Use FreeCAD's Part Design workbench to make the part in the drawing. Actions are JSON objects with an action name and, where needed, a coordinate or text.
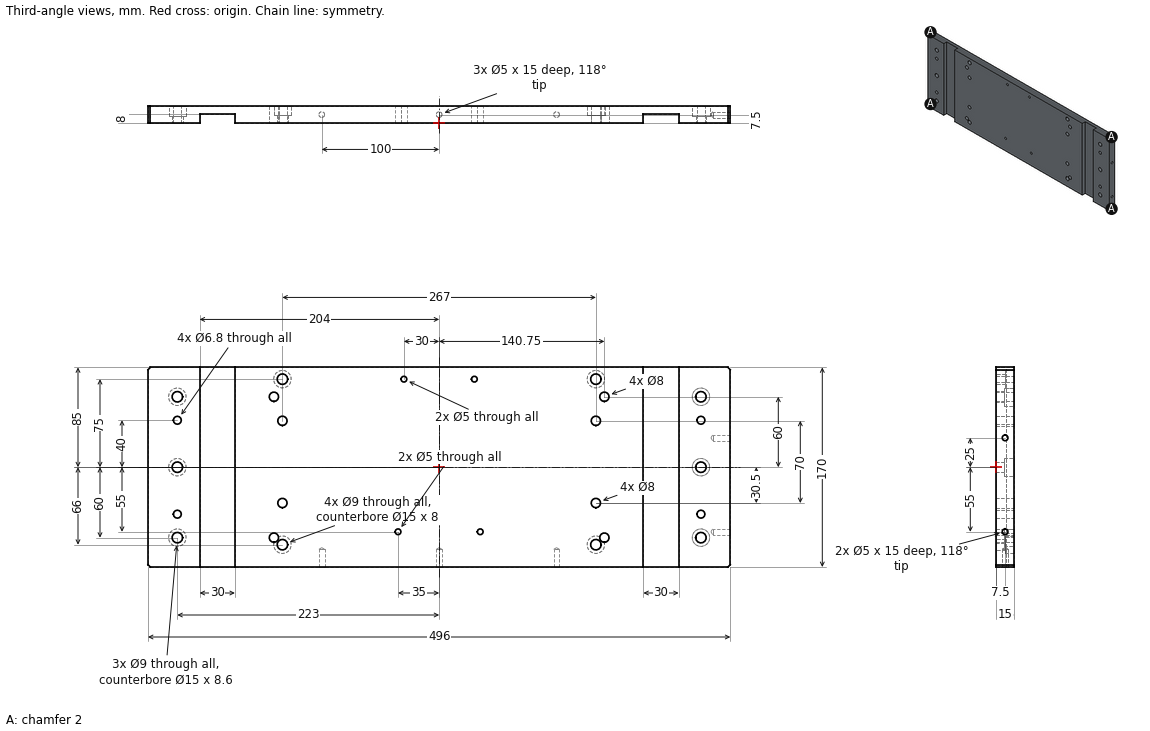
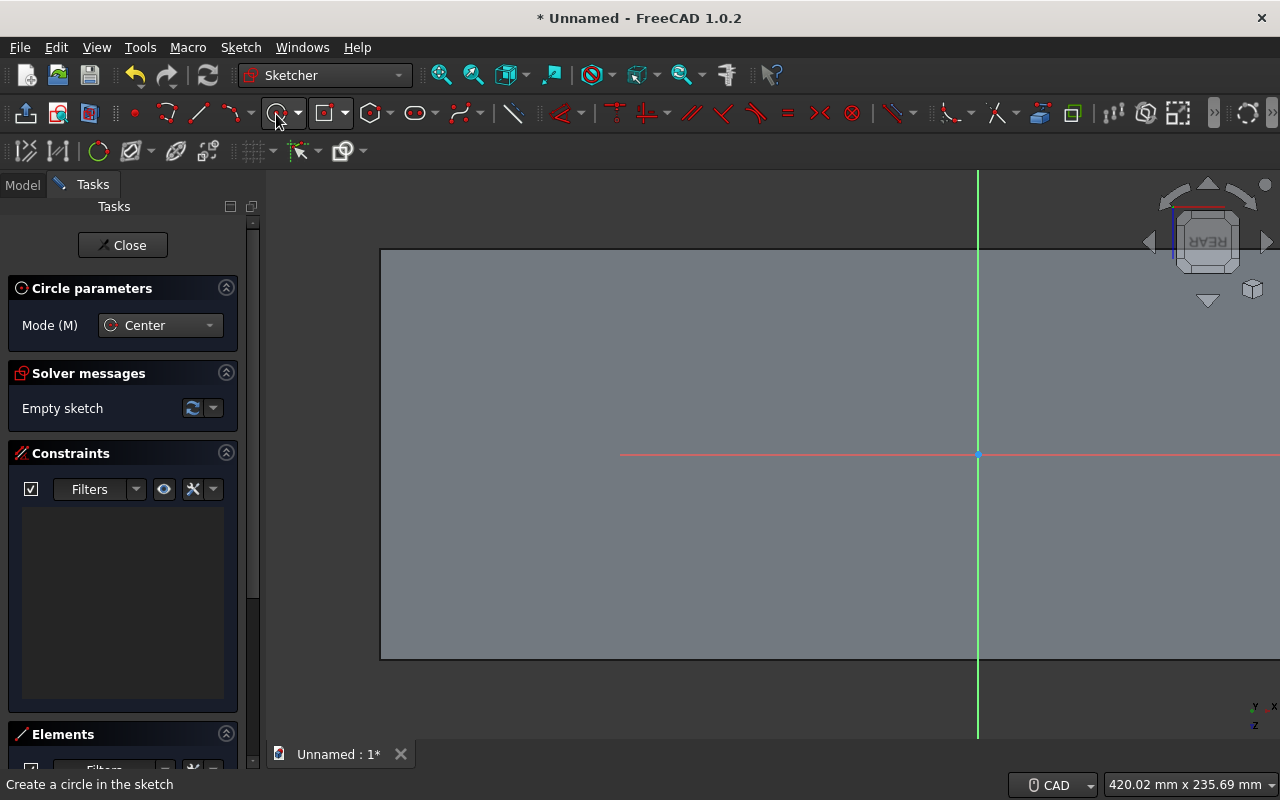
{"action": "scroll", "coordinate": [440, 310], "scroll_direction": "up", "scroll_amount": 4}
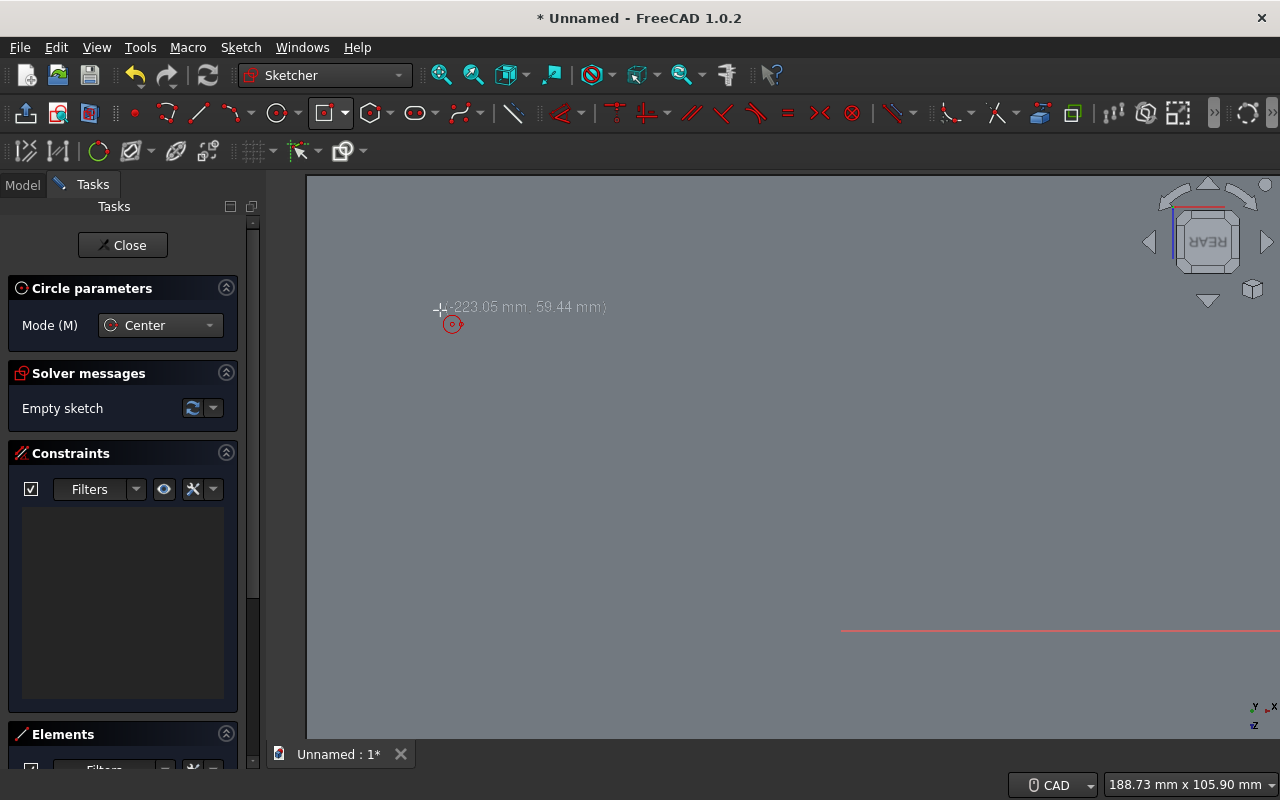
{"action": "left_click", "coordinate": [440, 309]}
{"action": "mouse_move", "coordinate": [457, 292]}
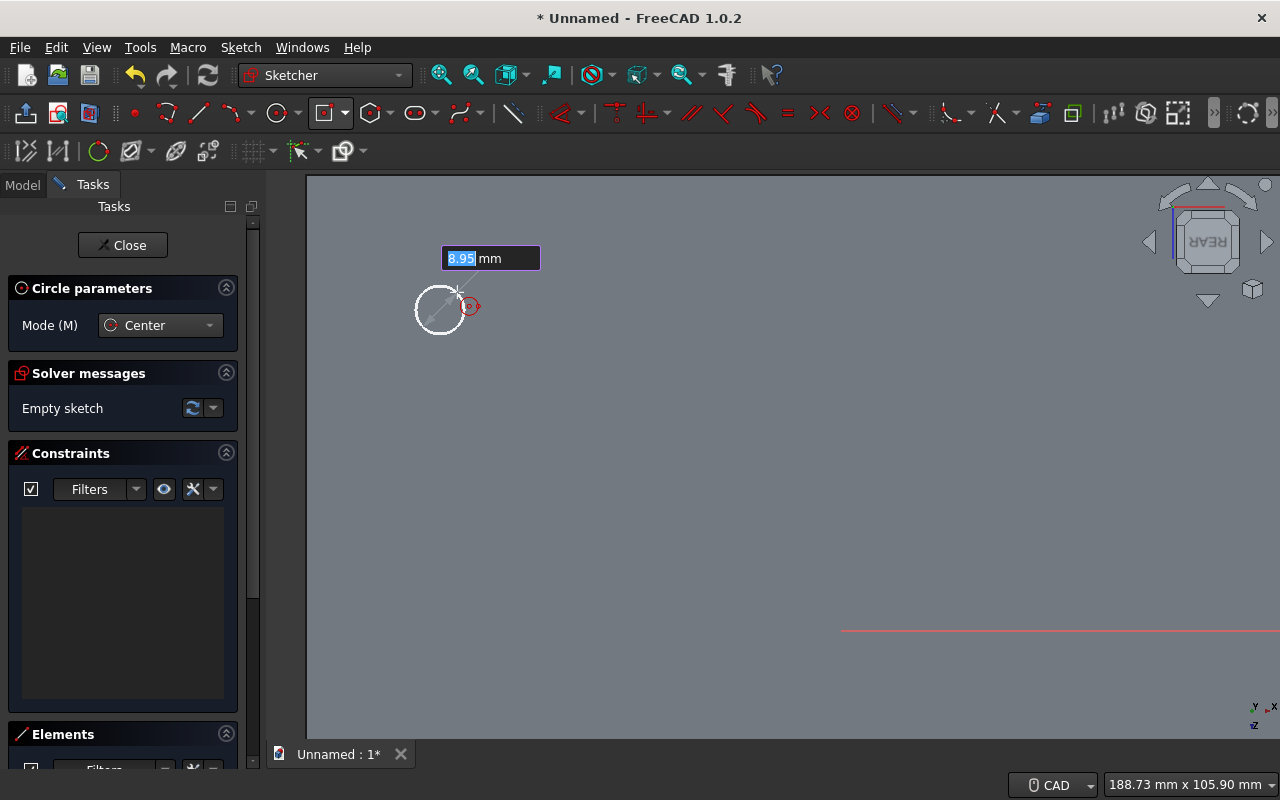
{"action": "type", "text": "9"}
{"action": "key", "text": "Return"}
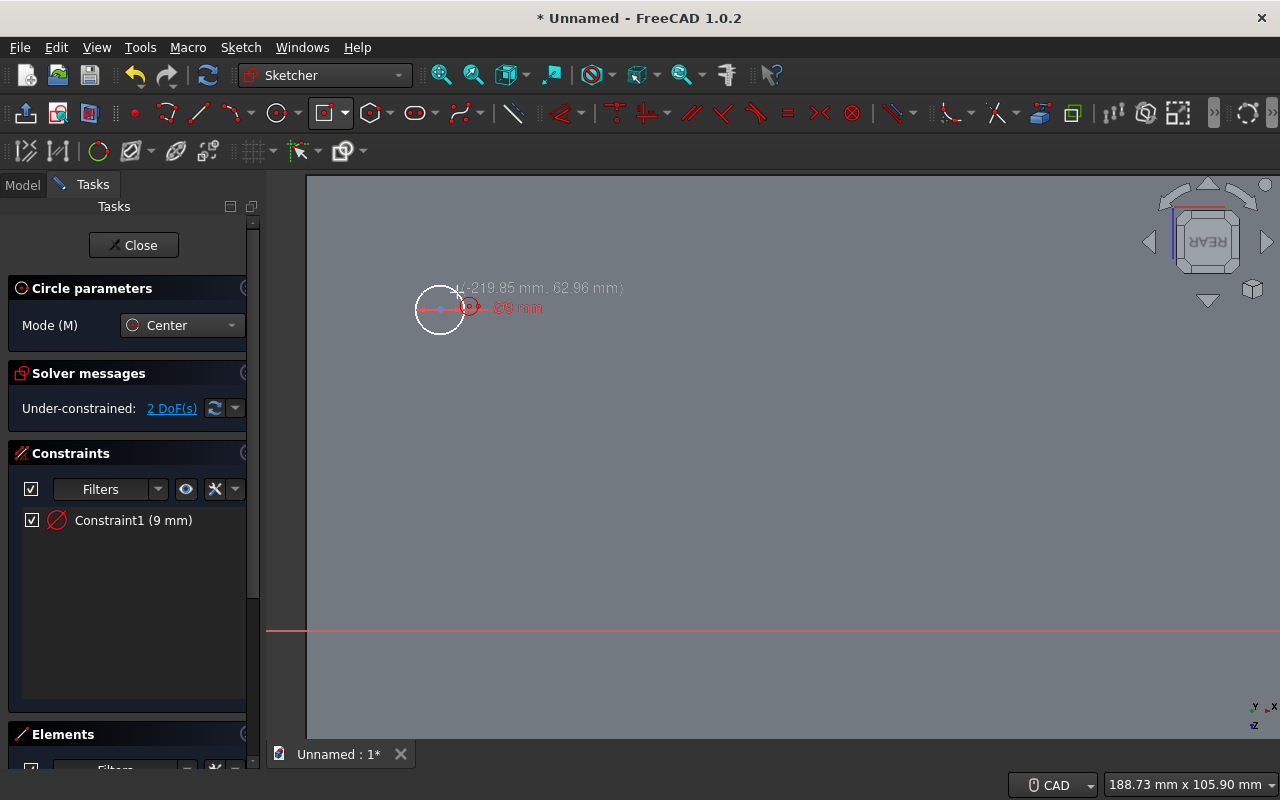
{"action": "left_click", "coordinate": [440, 631]}
{"action": "mouse_move", "coordinate": [457, 614]}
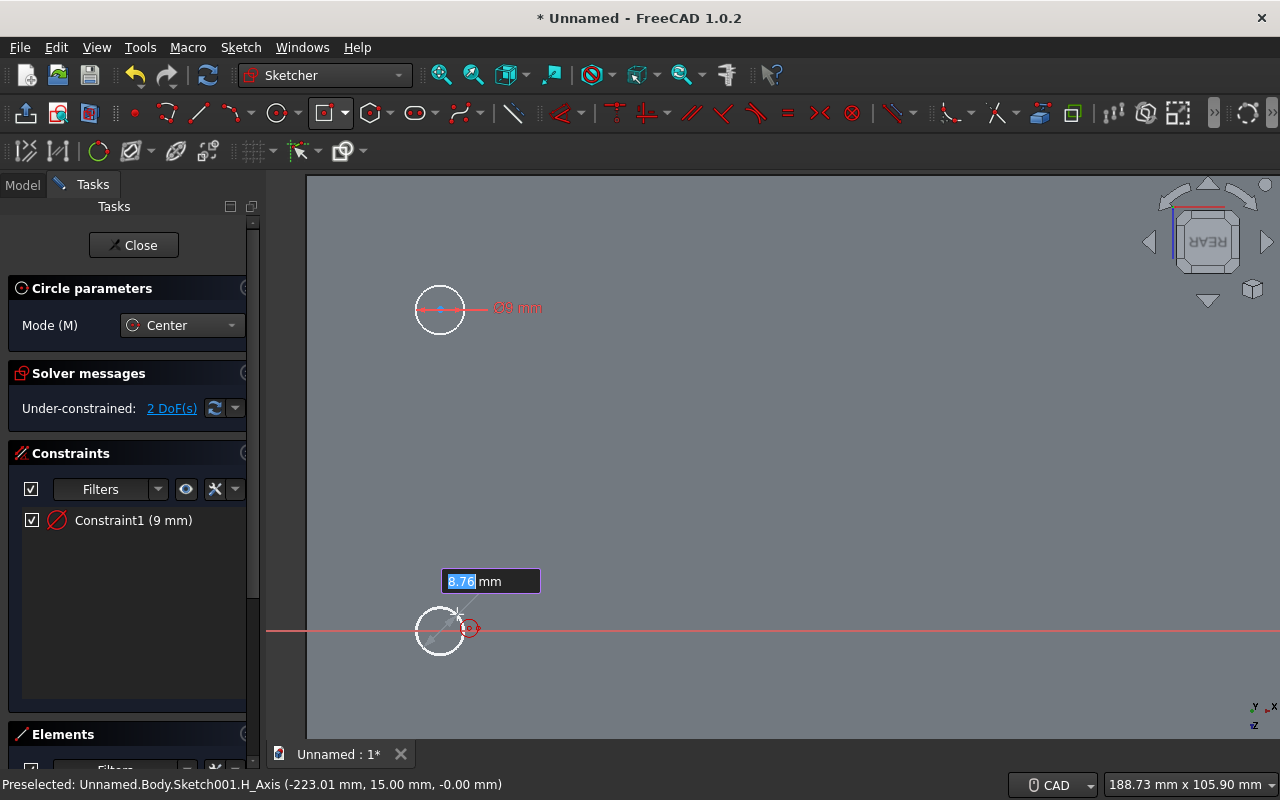
{"action": "type", "text": "9"}
{"action": "key", "text": "Return"}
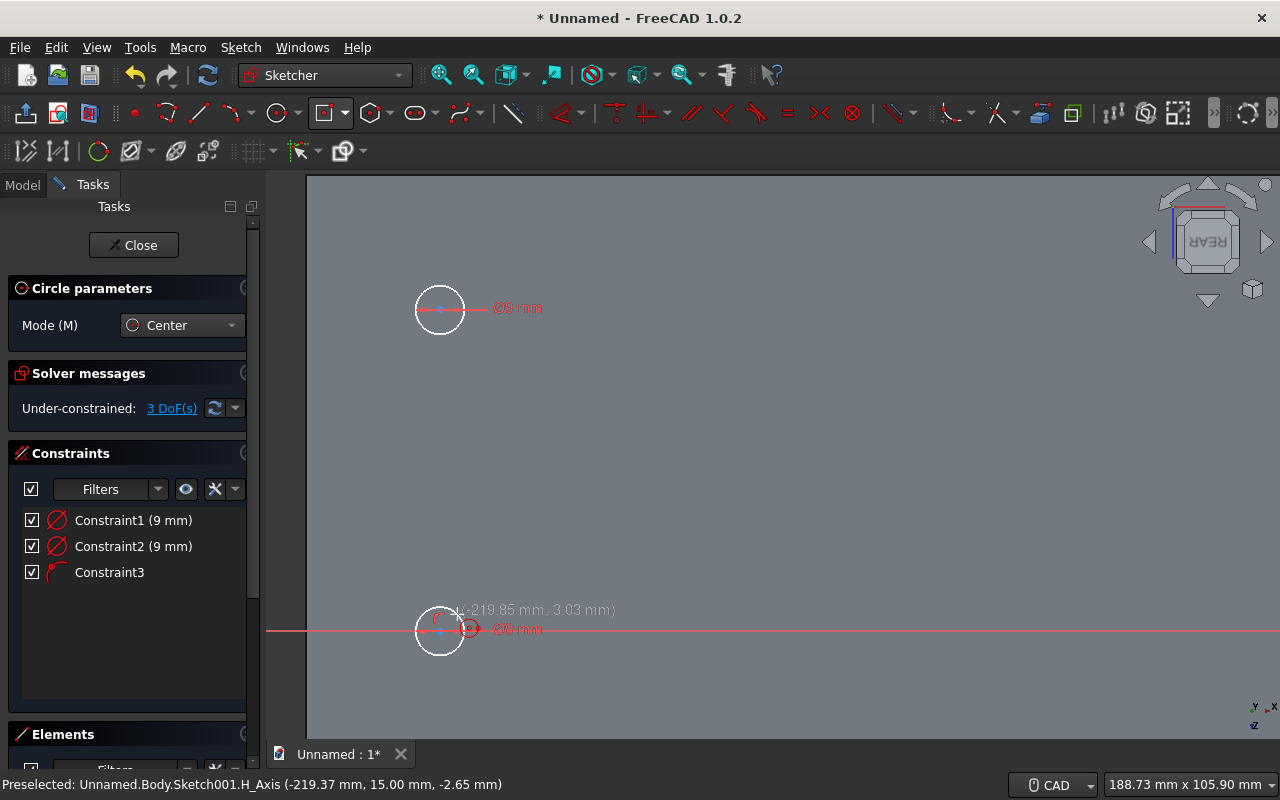
{"action": "scroll", "coordinate": [441, 310], "scroll_direction": "down", "scroll_amount": 4}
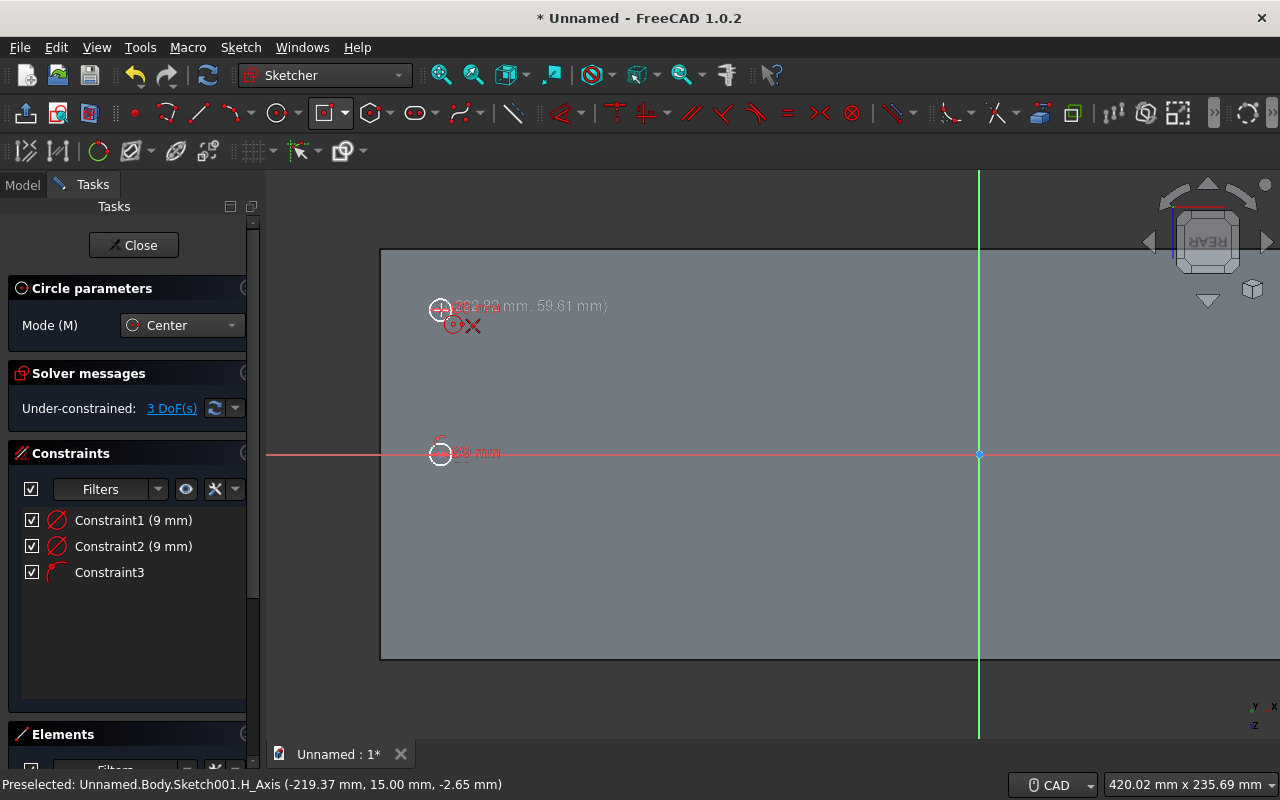
{"action": "scroll", "coordinate": [441, 599], "scroll_direction": "up", "scroll_amount": 4}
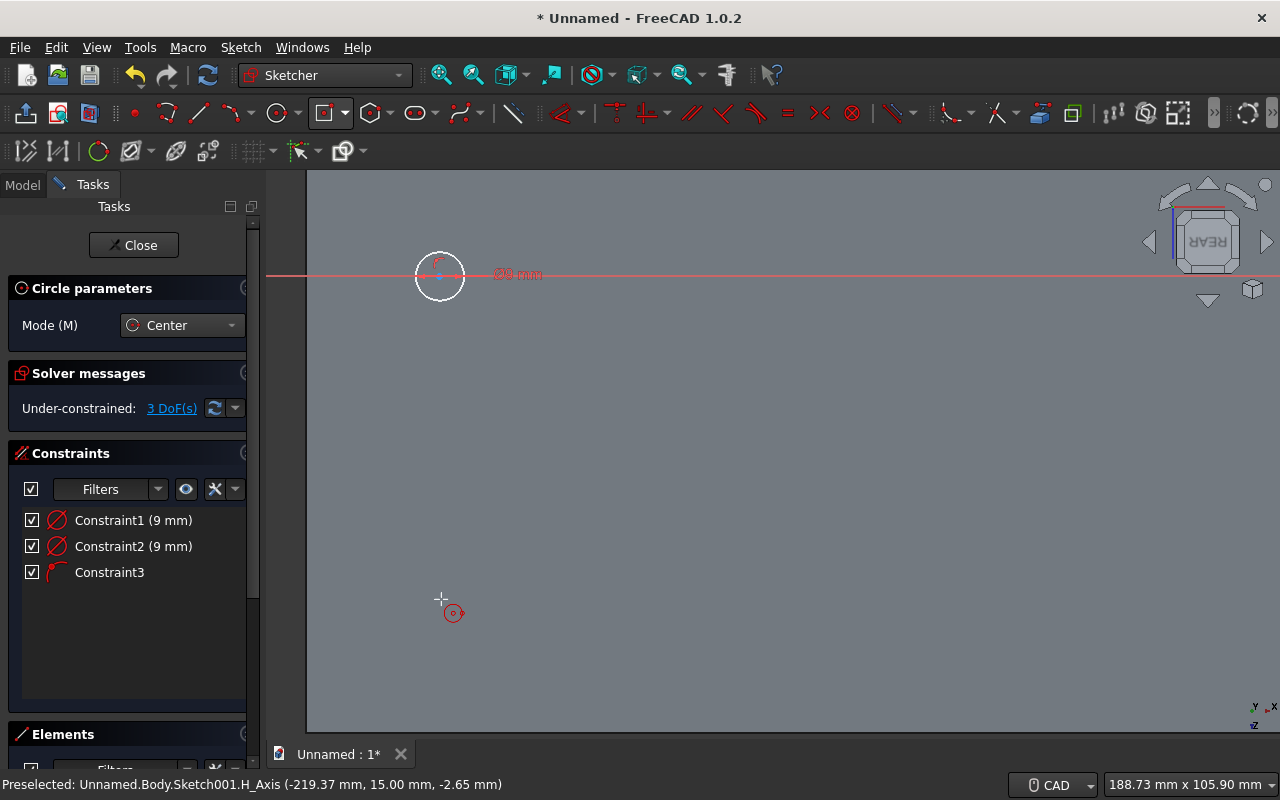
{"action": "left_click", "coordinate": [440, 599]}
{"action": "mouse_move", "coordinate": [457, 582]}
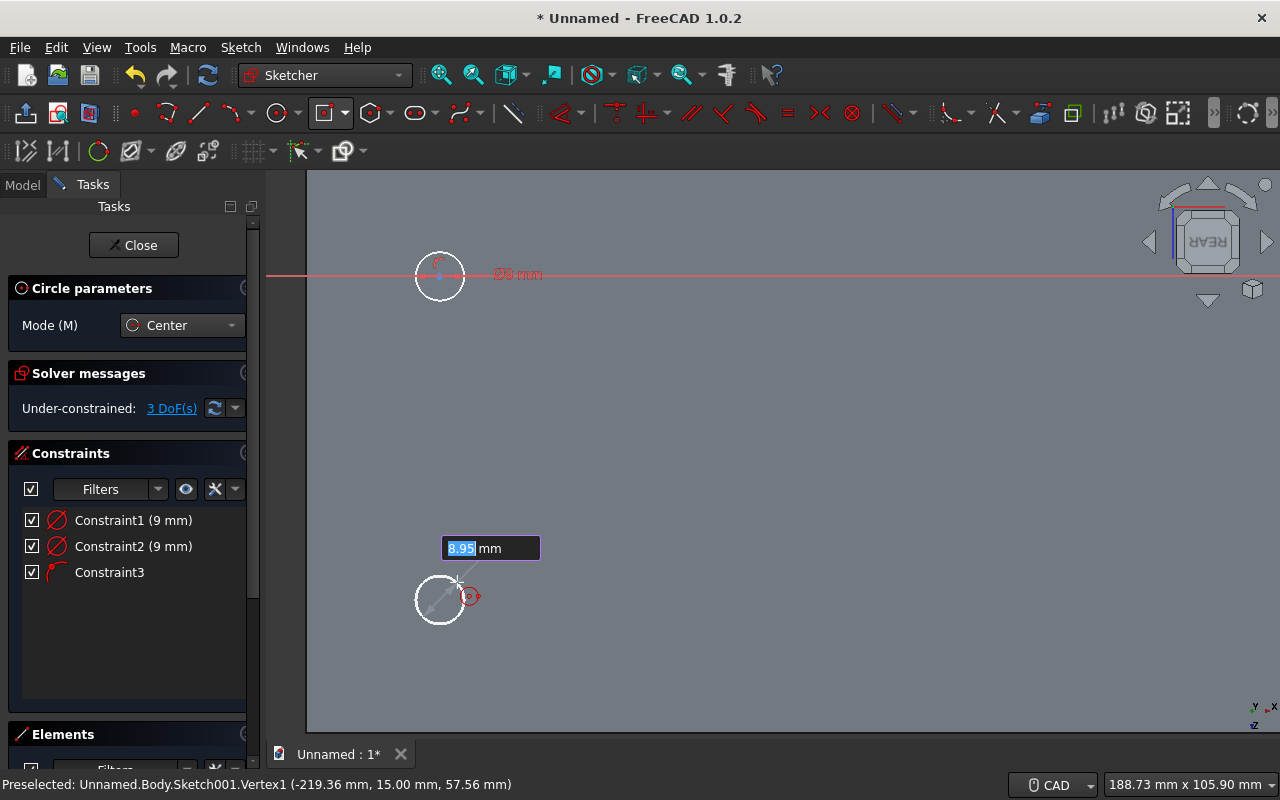
{"action": "type", "text": "9"}
{"action": "key", "text": "Return"}
{"action": "key", "text": "Escape"}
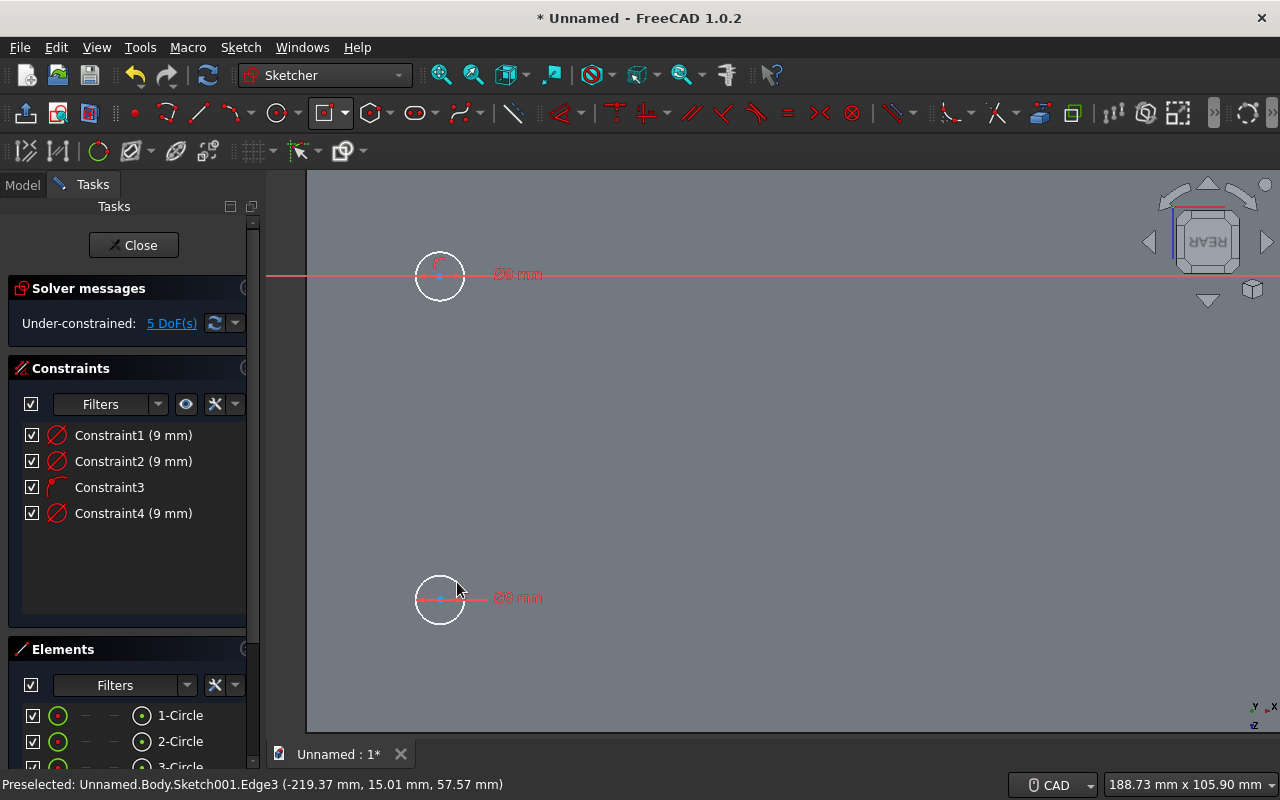
{"action": "scroll", "coordinate": [441, 600], "scroll_direction": "down", "scroll_amount": 4}